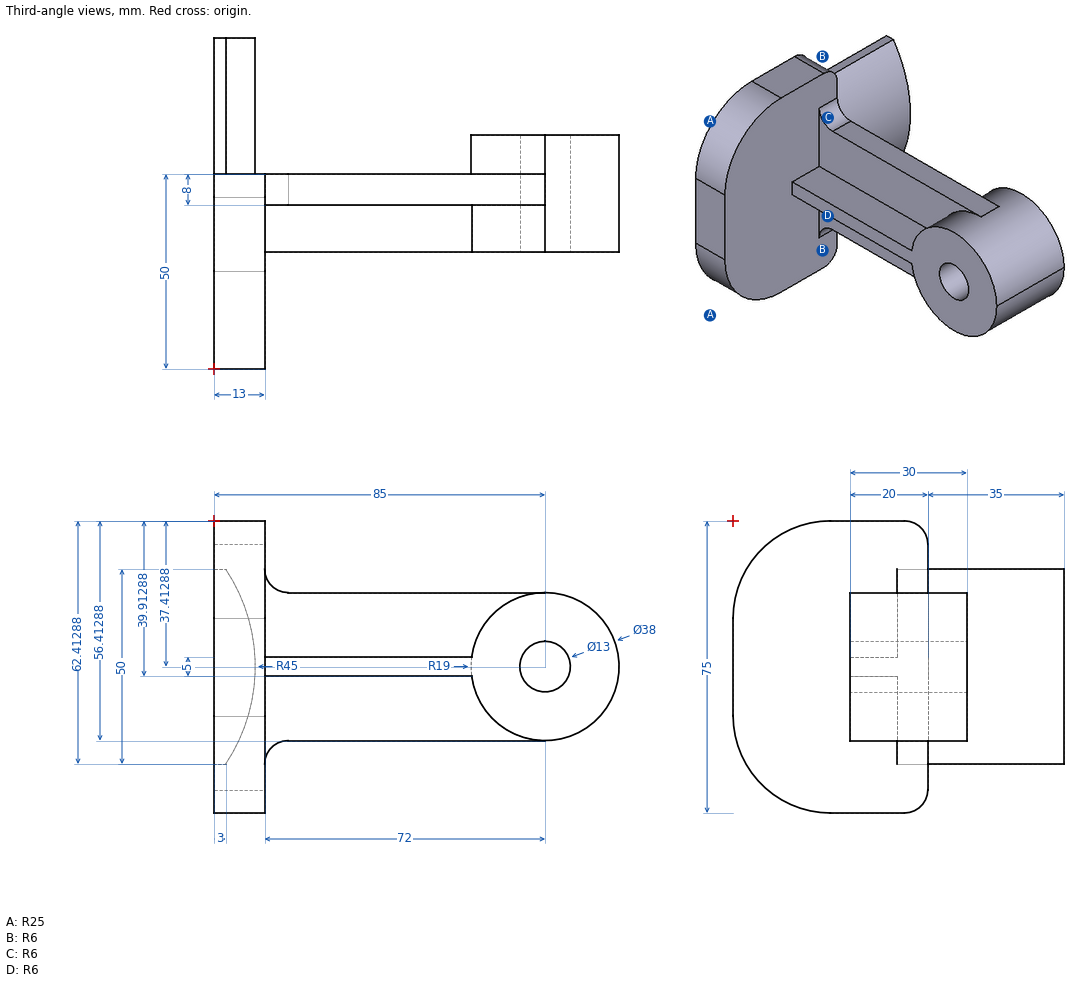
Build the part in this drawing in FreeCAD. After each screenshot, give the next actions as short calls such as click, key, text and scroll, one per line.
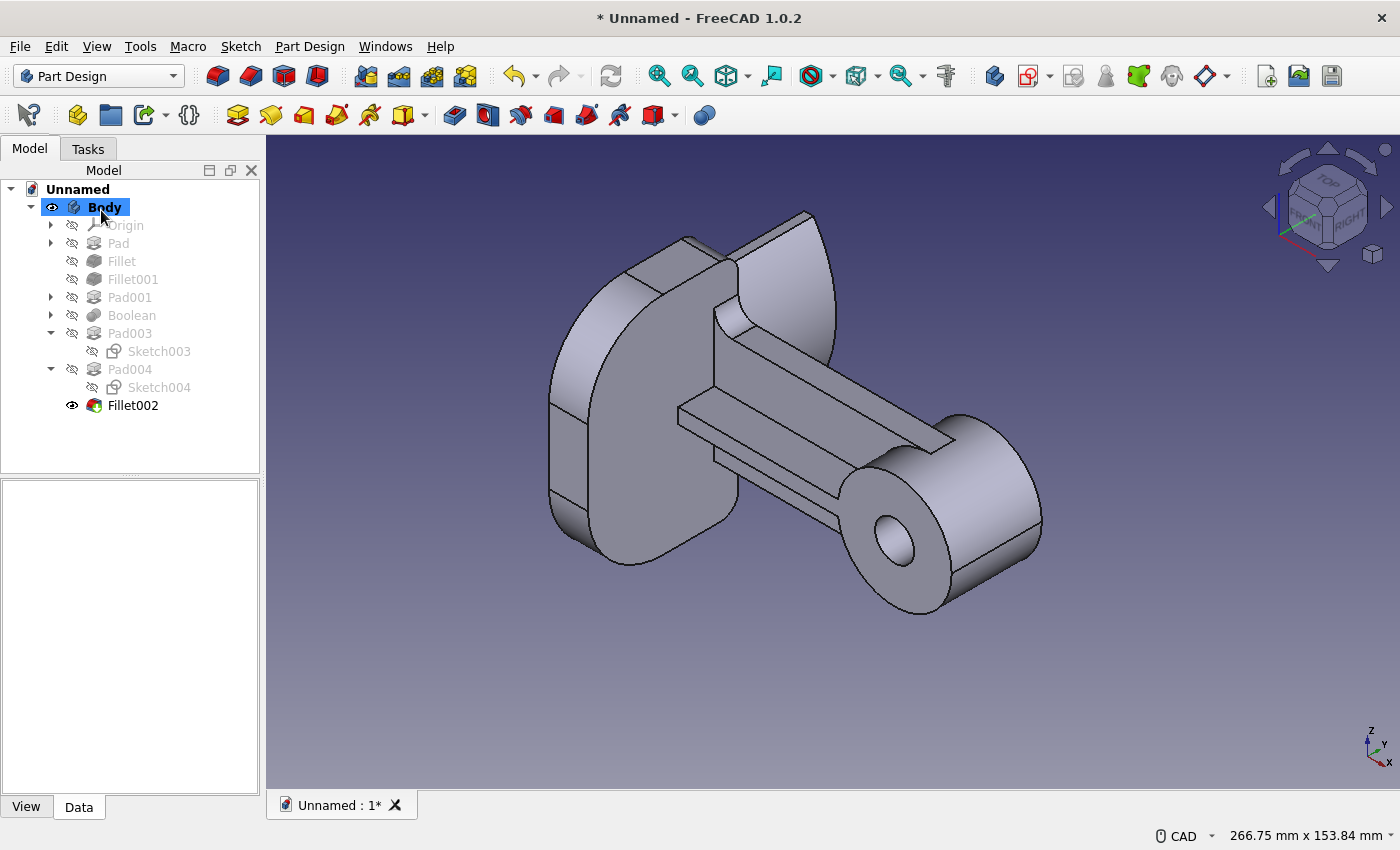
key(2)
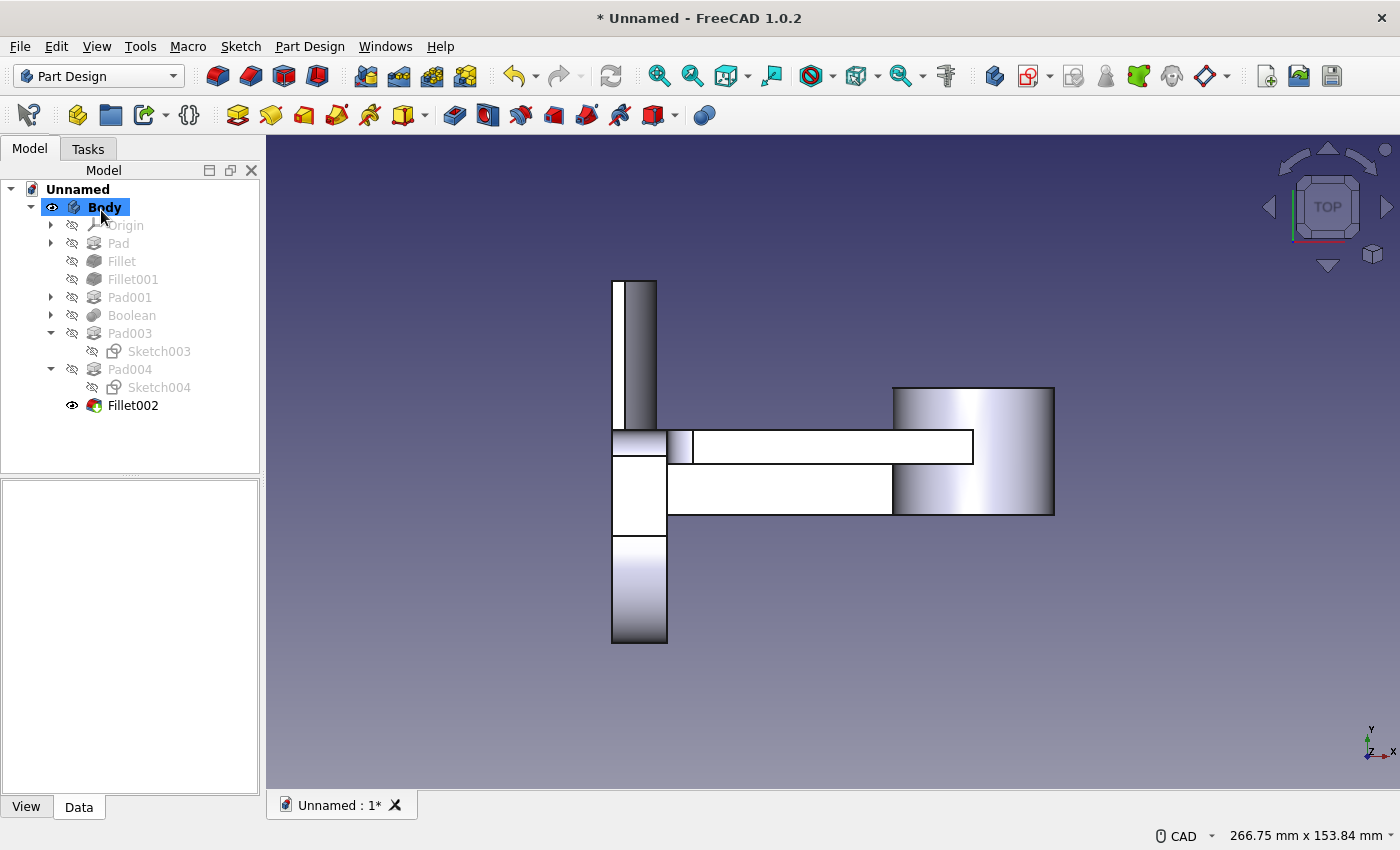
key(0)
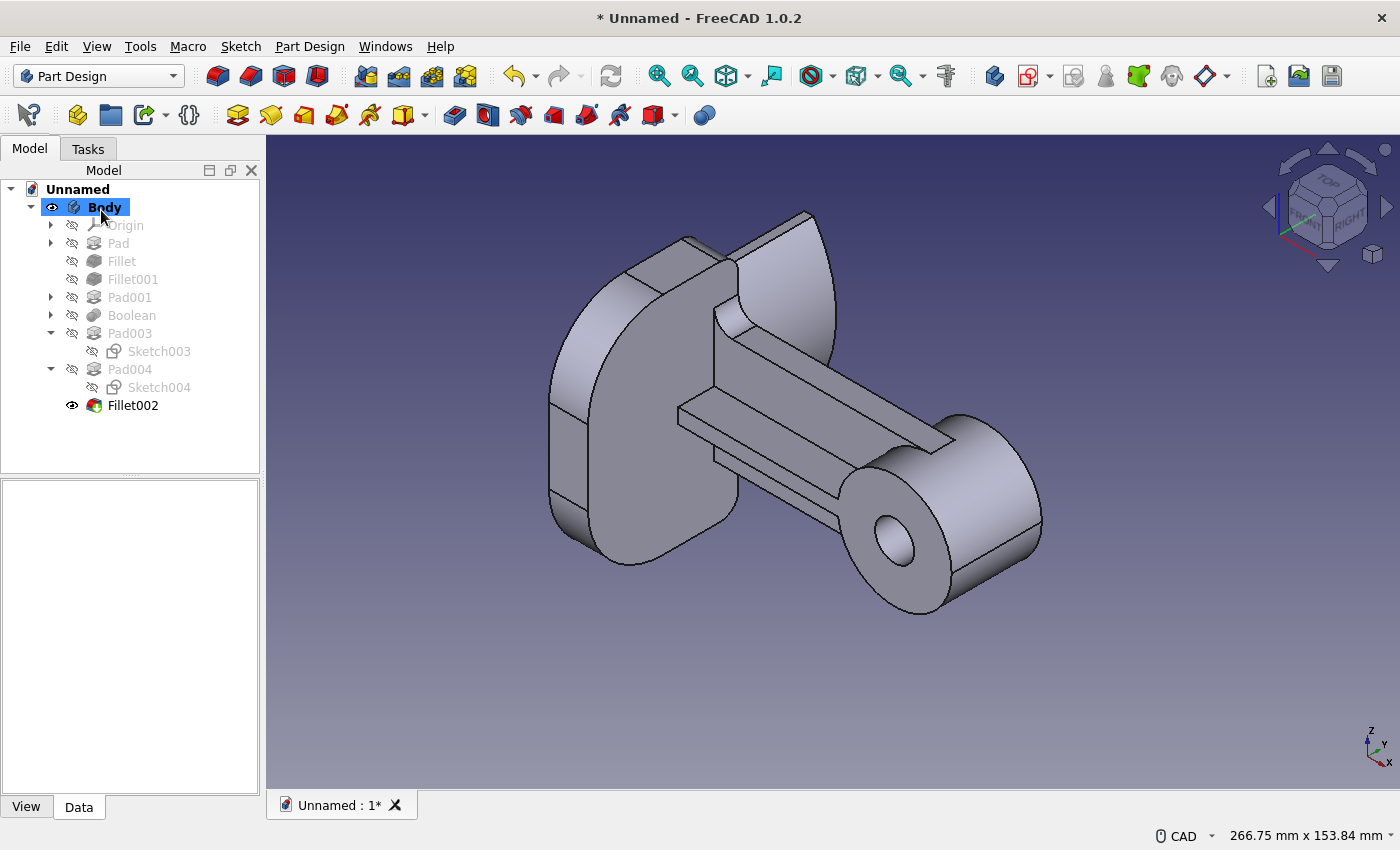
key(1)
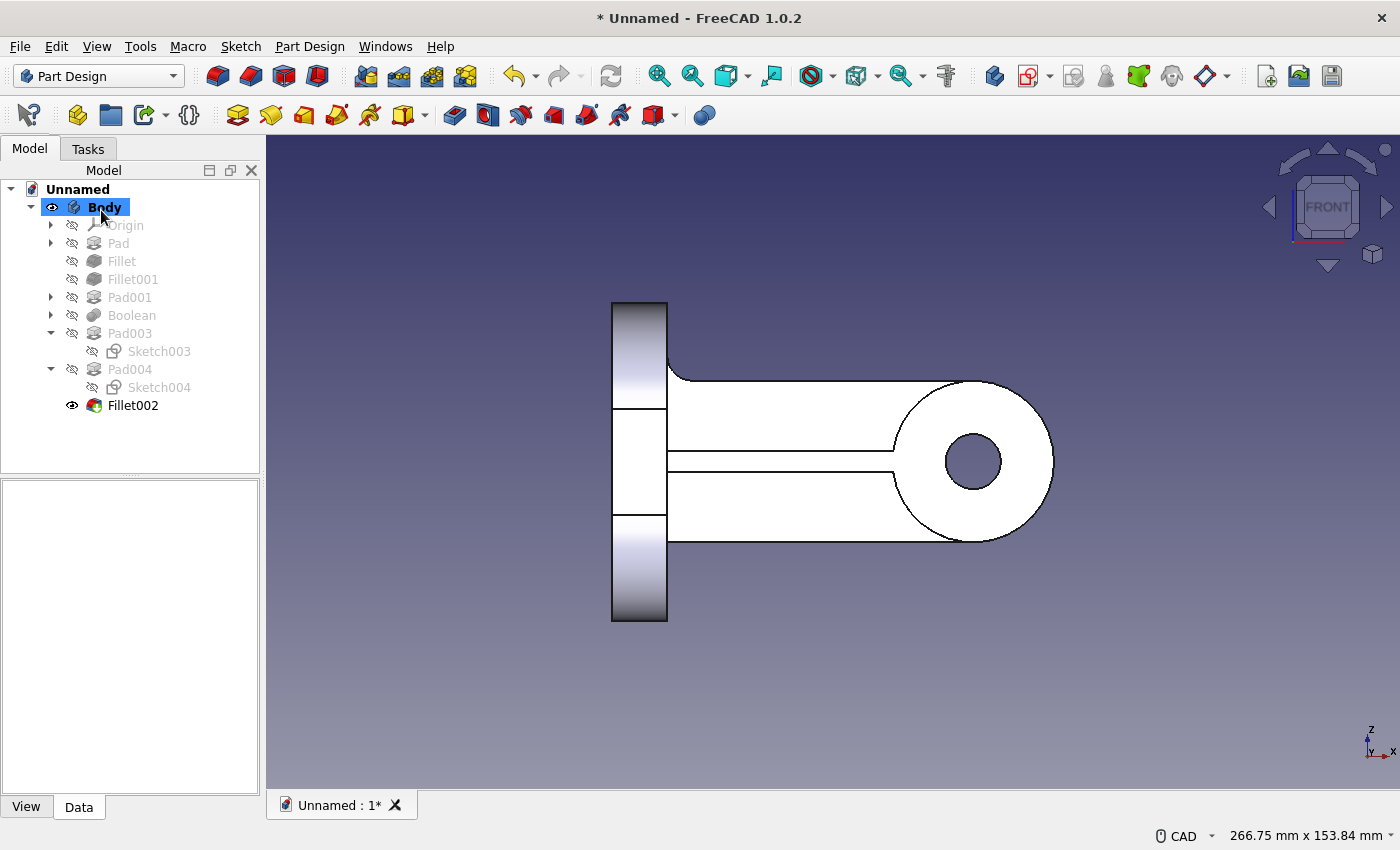
key(3)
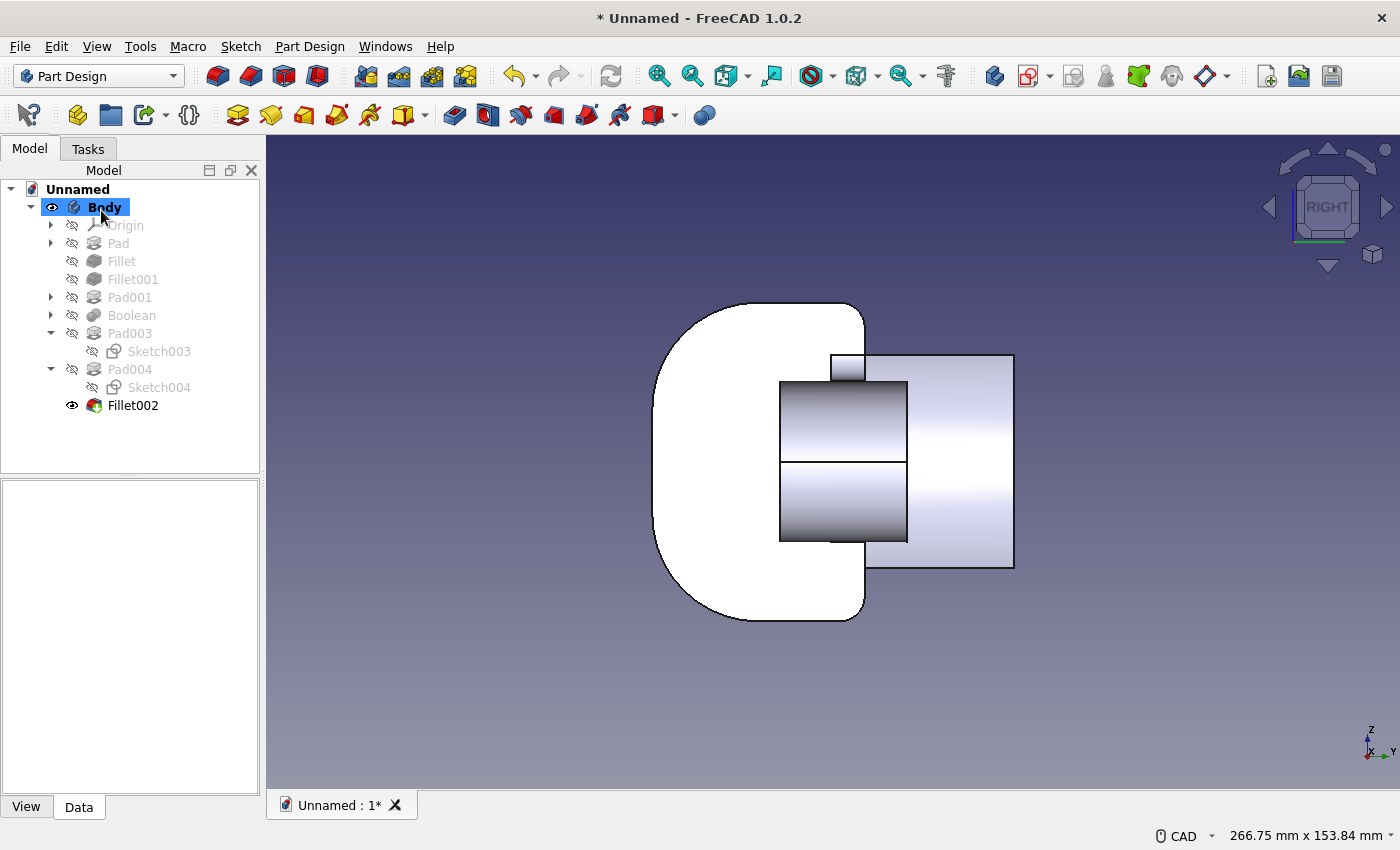
key(5)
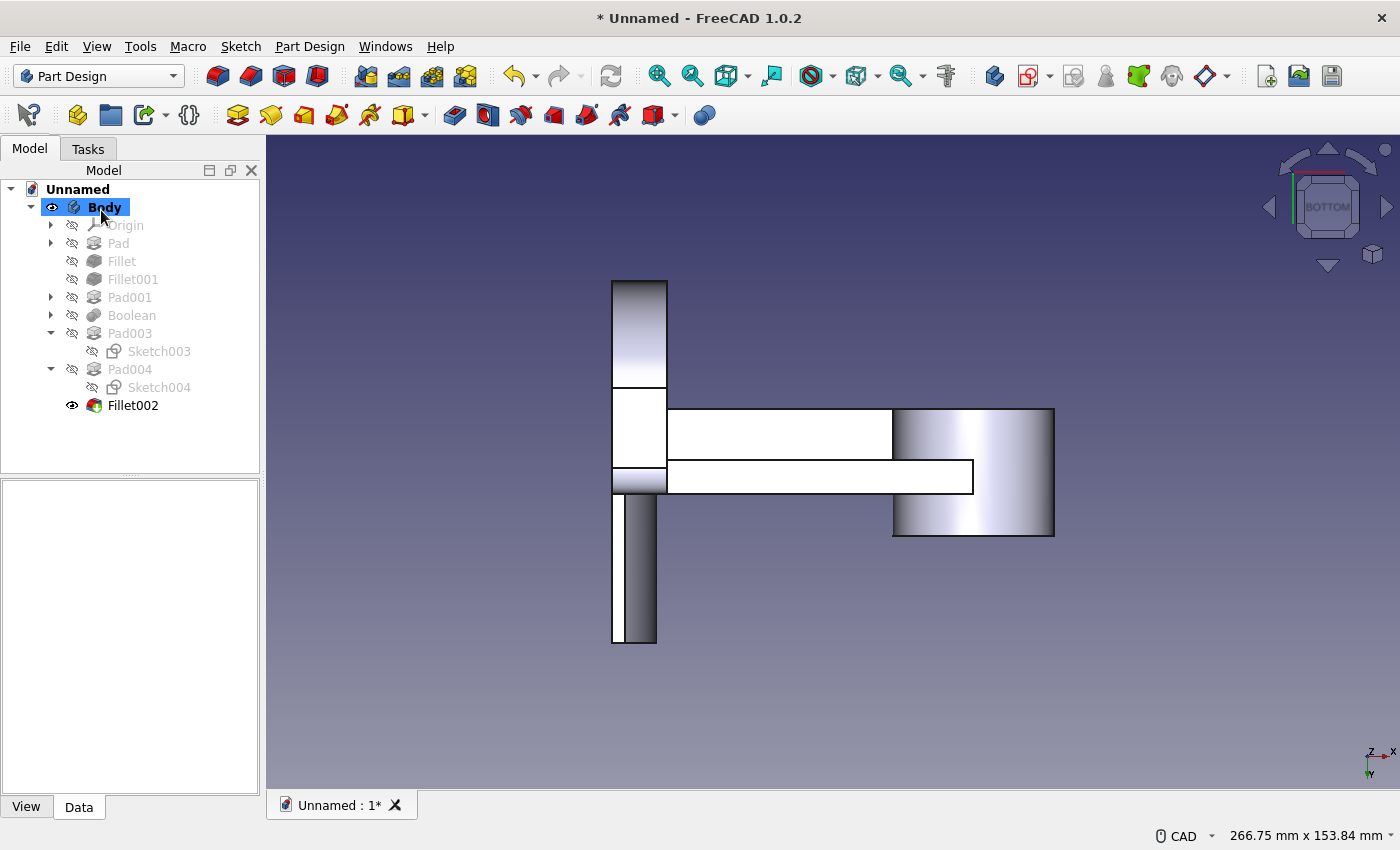
key(4)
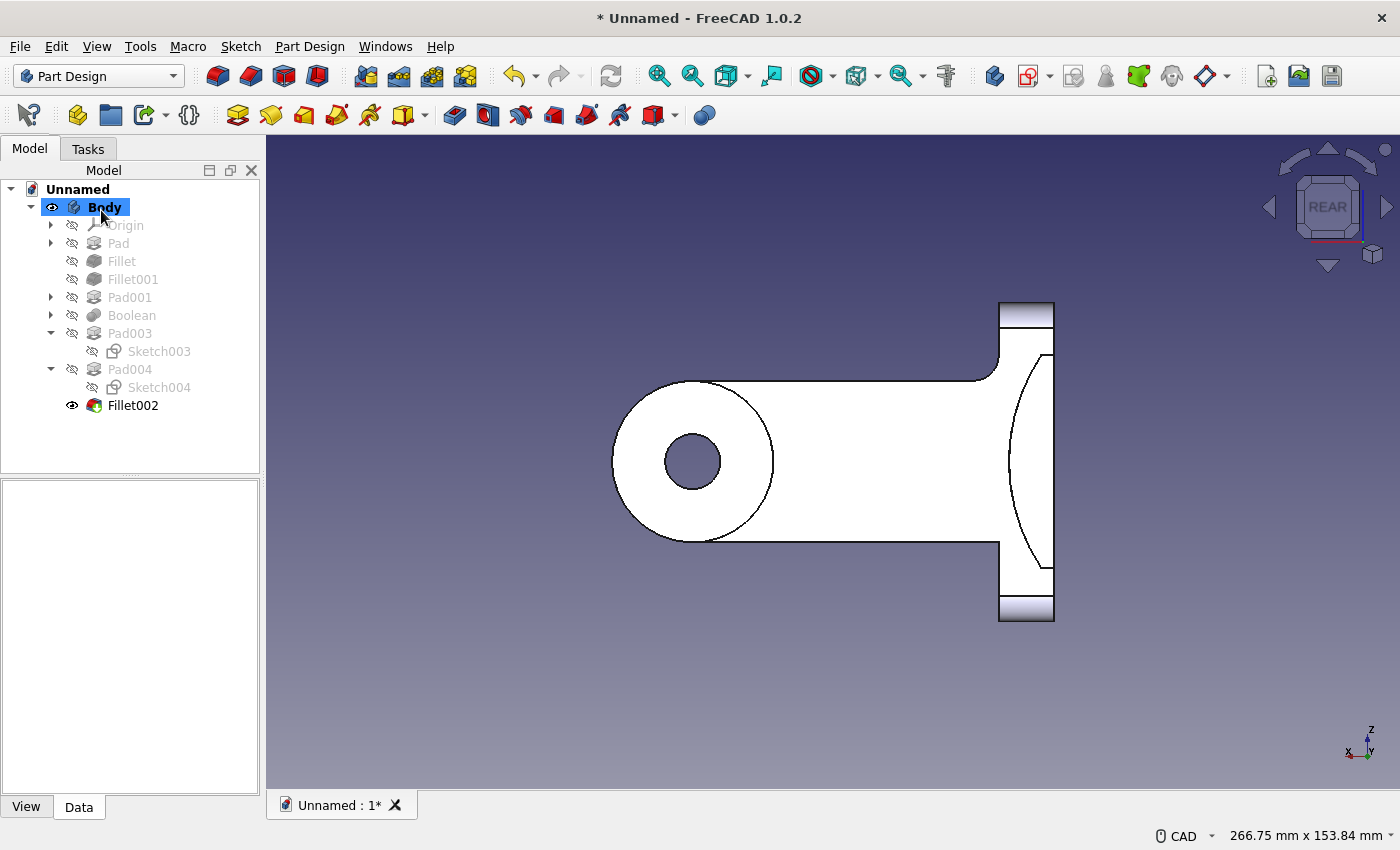
key(6)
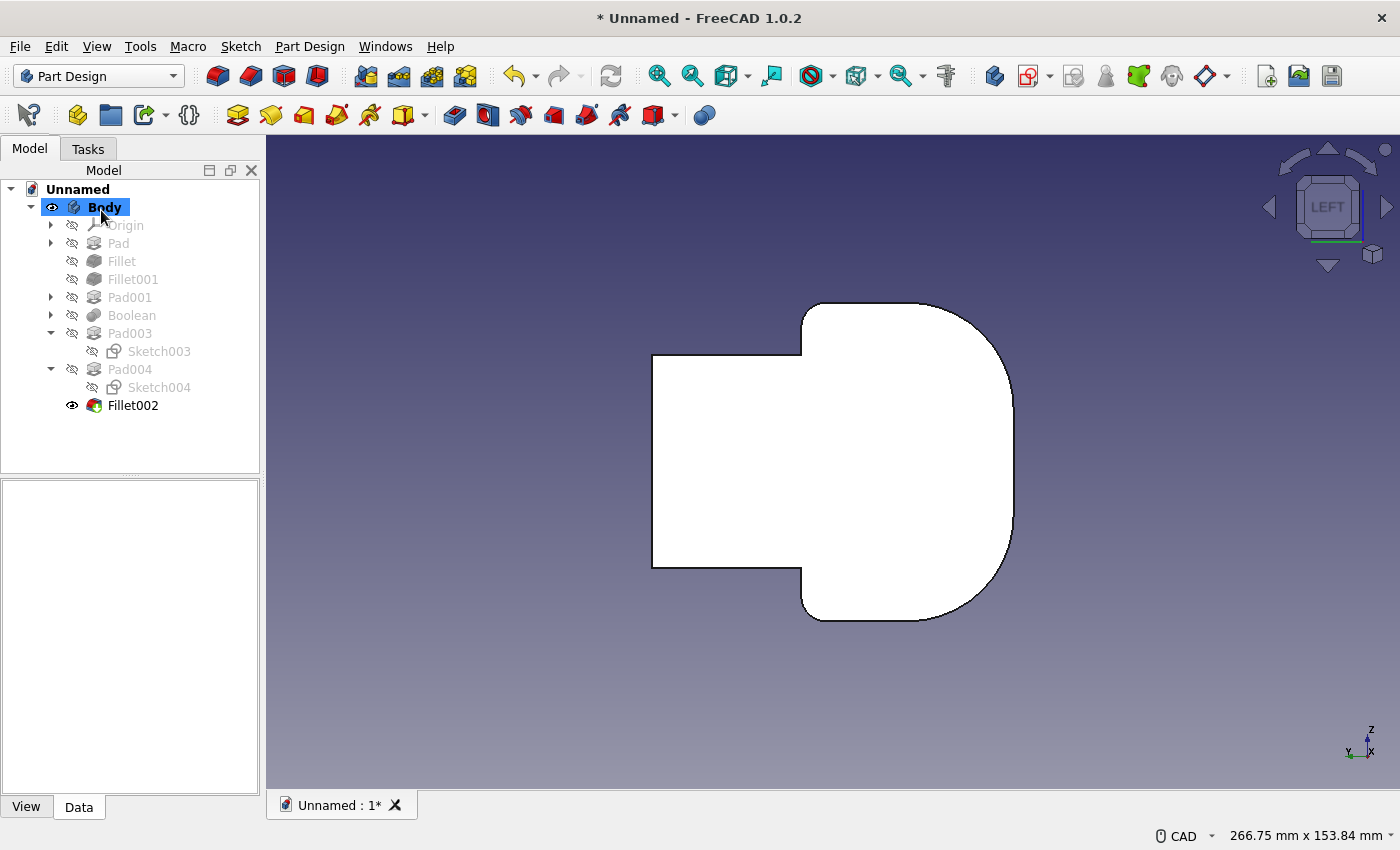
key(v)
key(3)